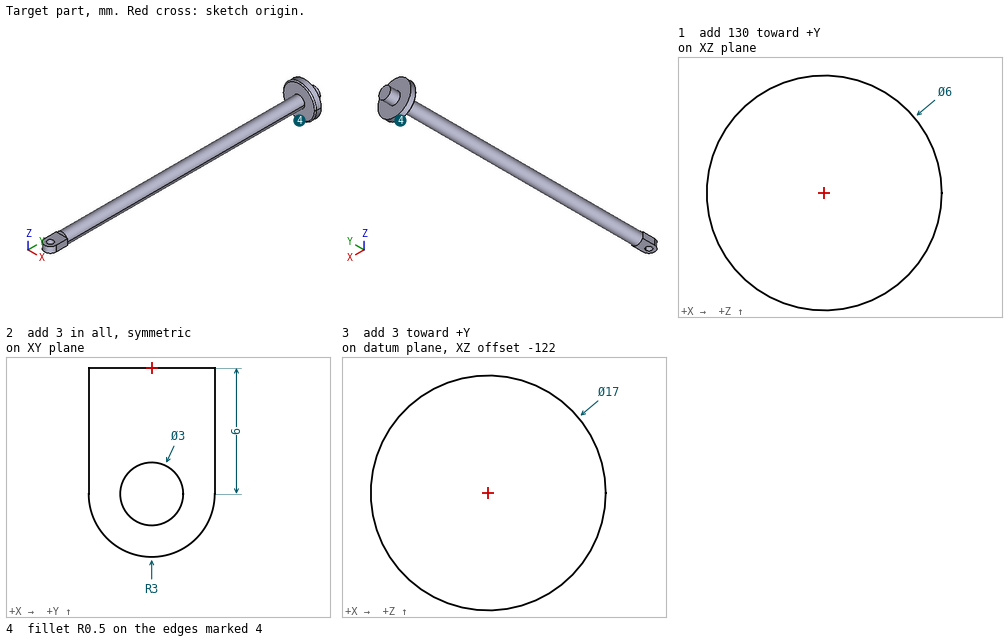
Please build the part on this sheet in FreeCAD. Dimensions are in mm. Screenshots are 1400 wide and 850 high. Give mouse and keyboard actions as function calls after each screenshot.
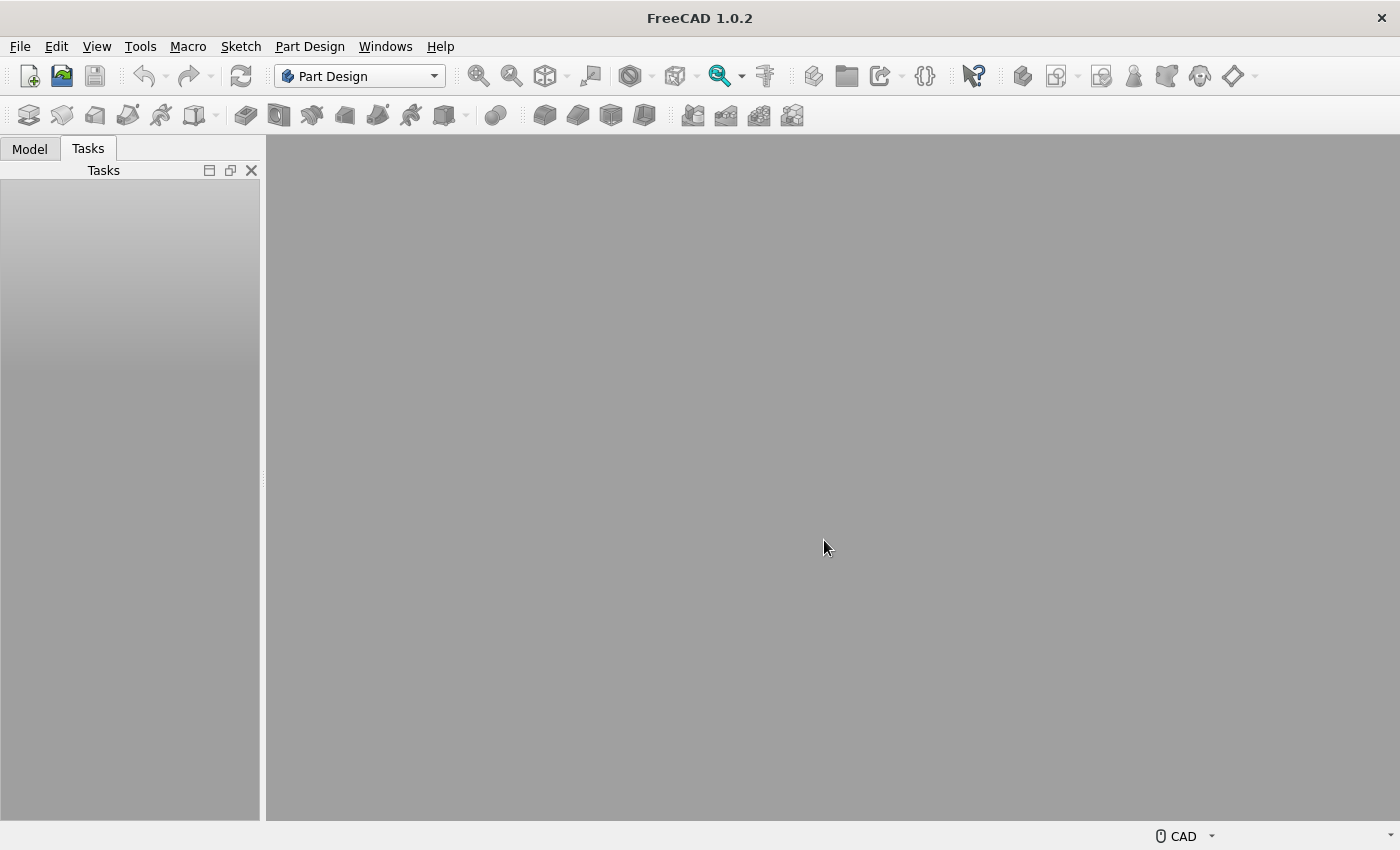
click(29, 76)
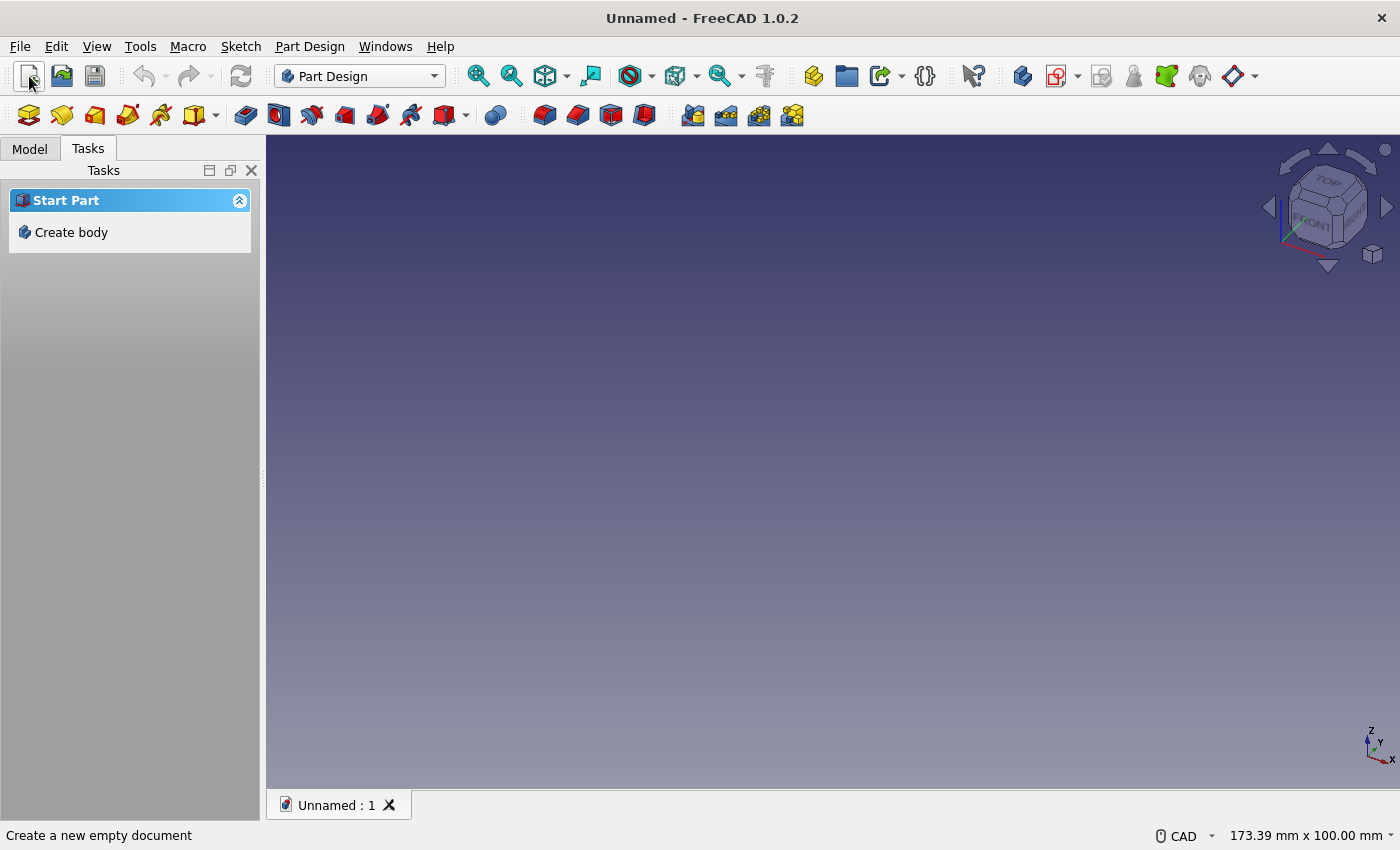
click(1056, 76)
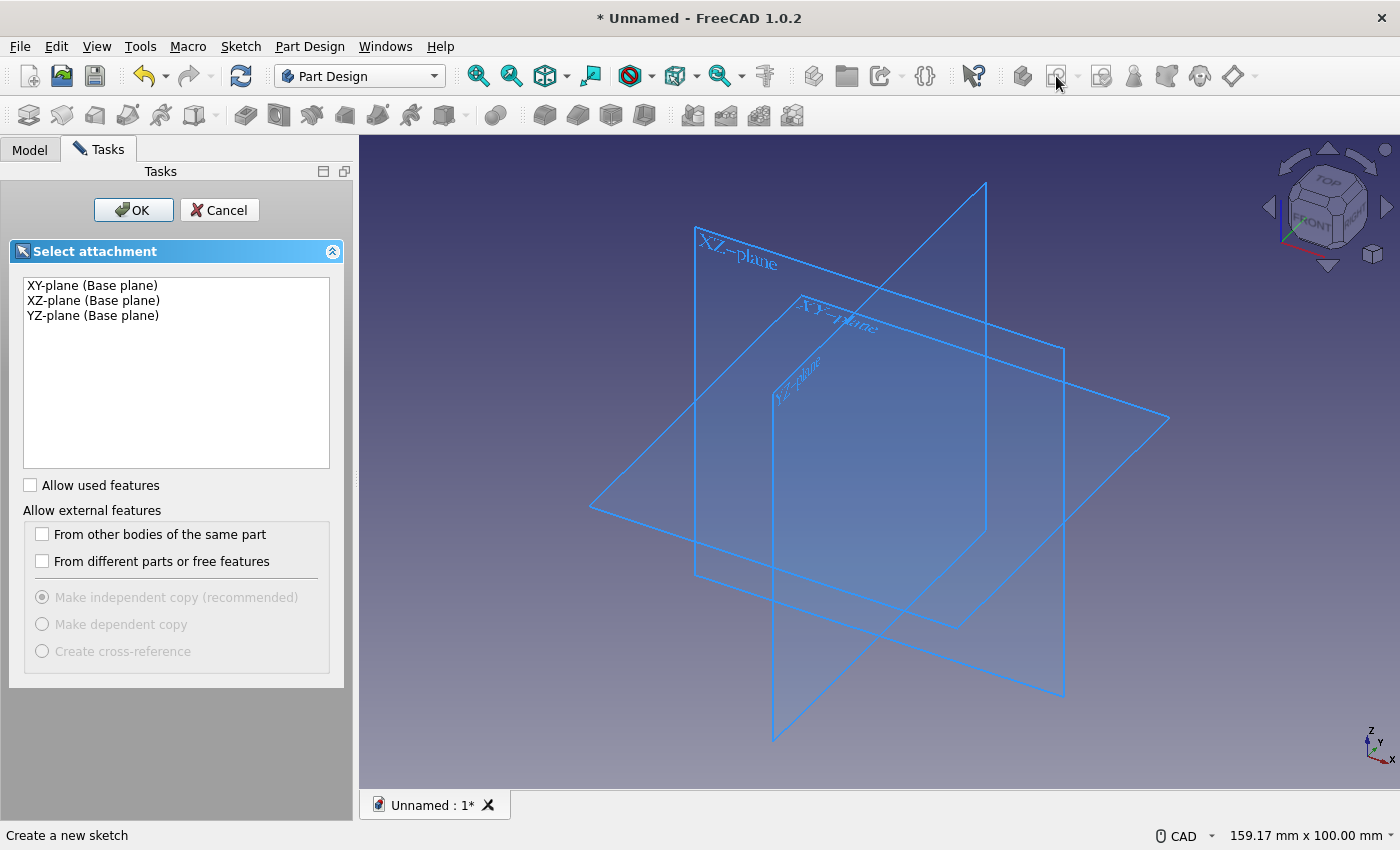
click(84, 300)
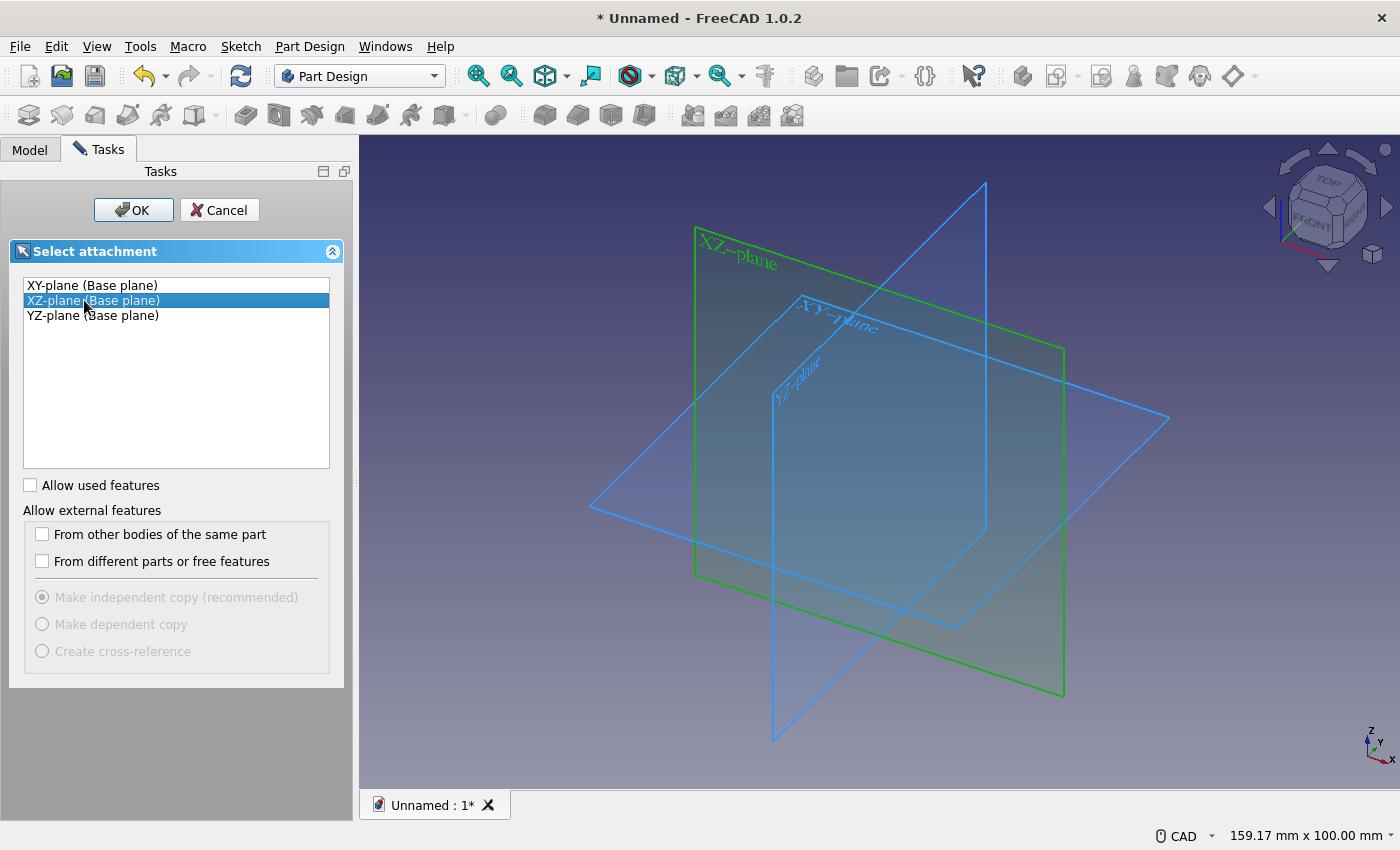
click(134, 210)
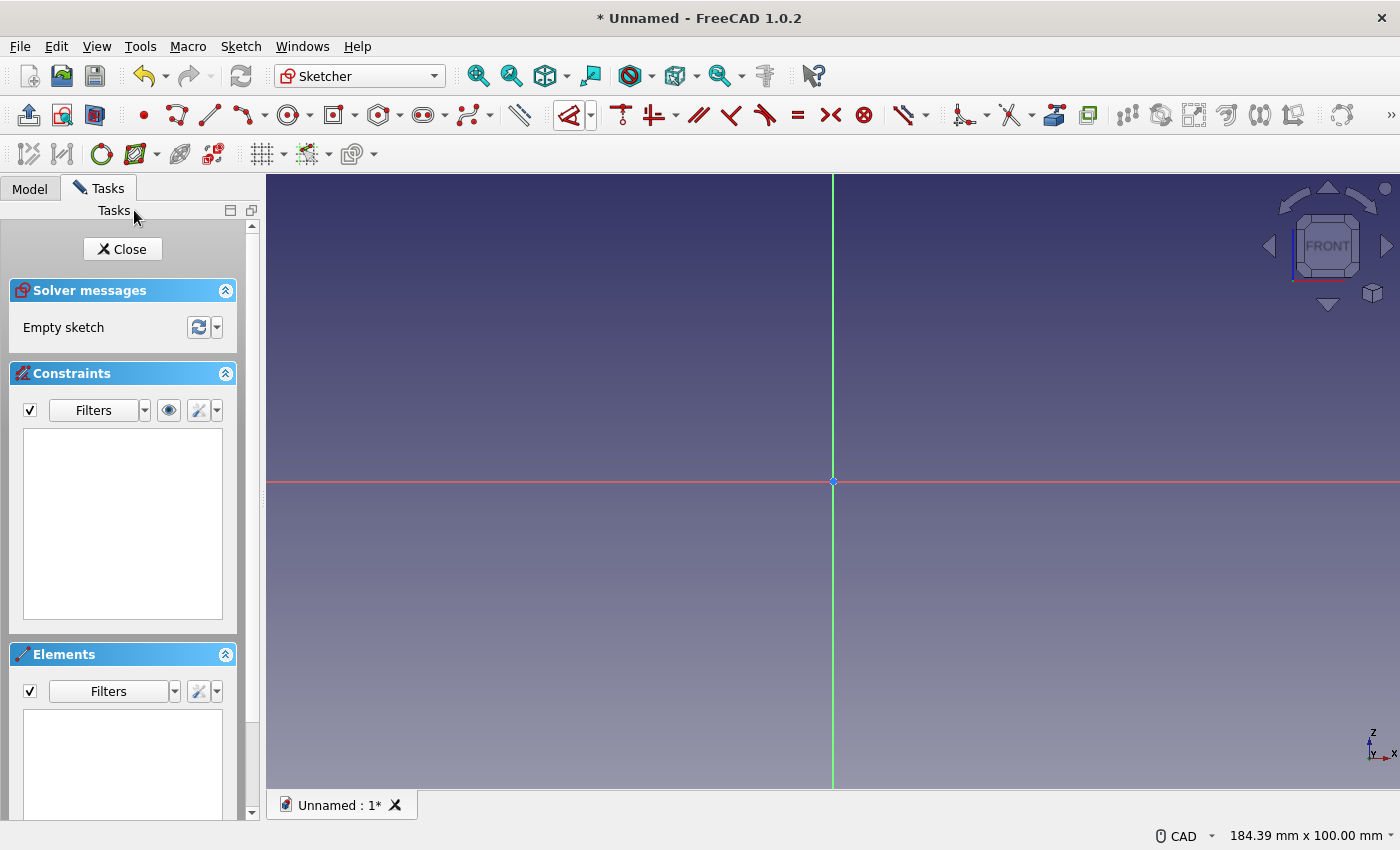
scroll(840, 482, up, 12)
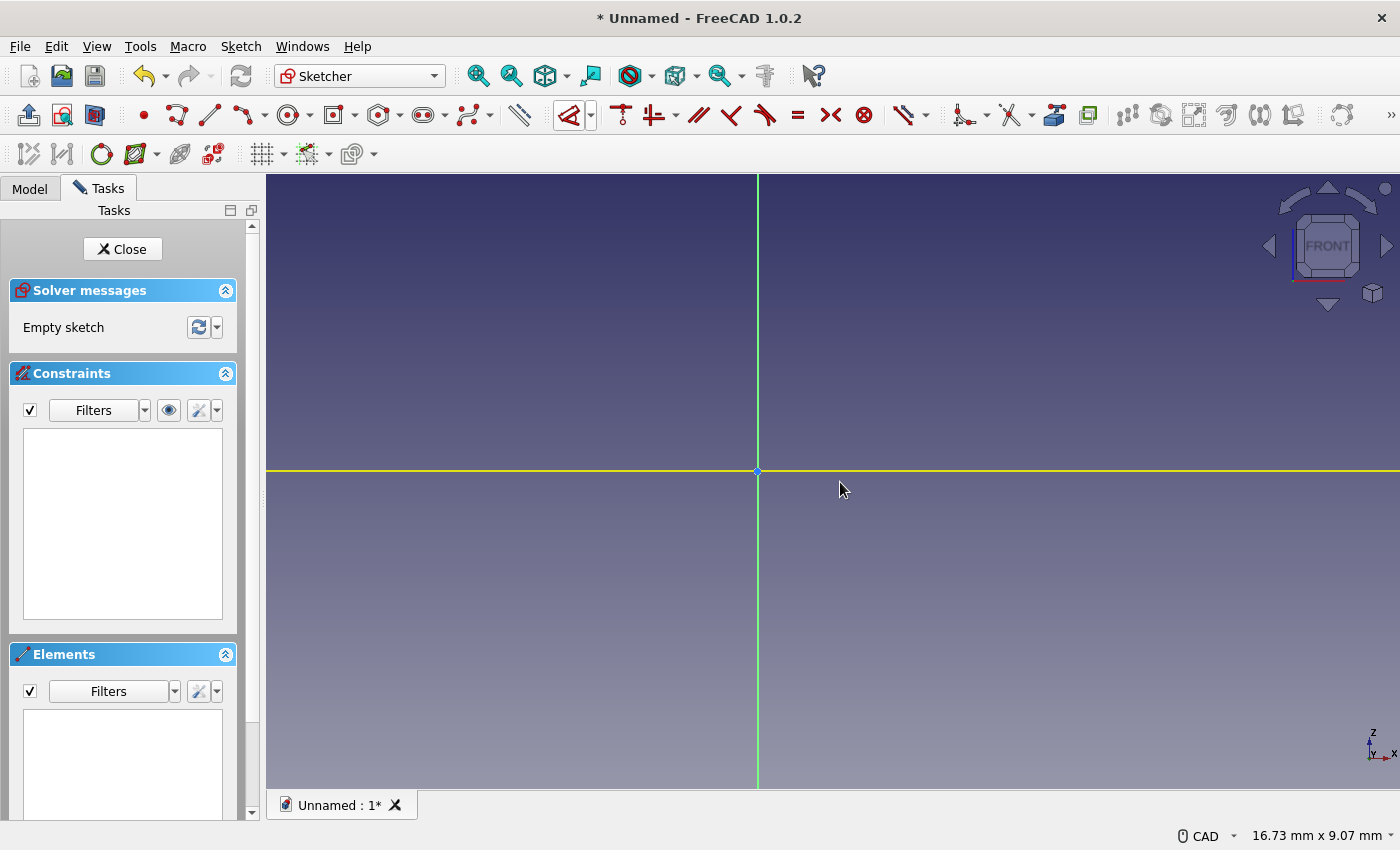
key(g)
key(c)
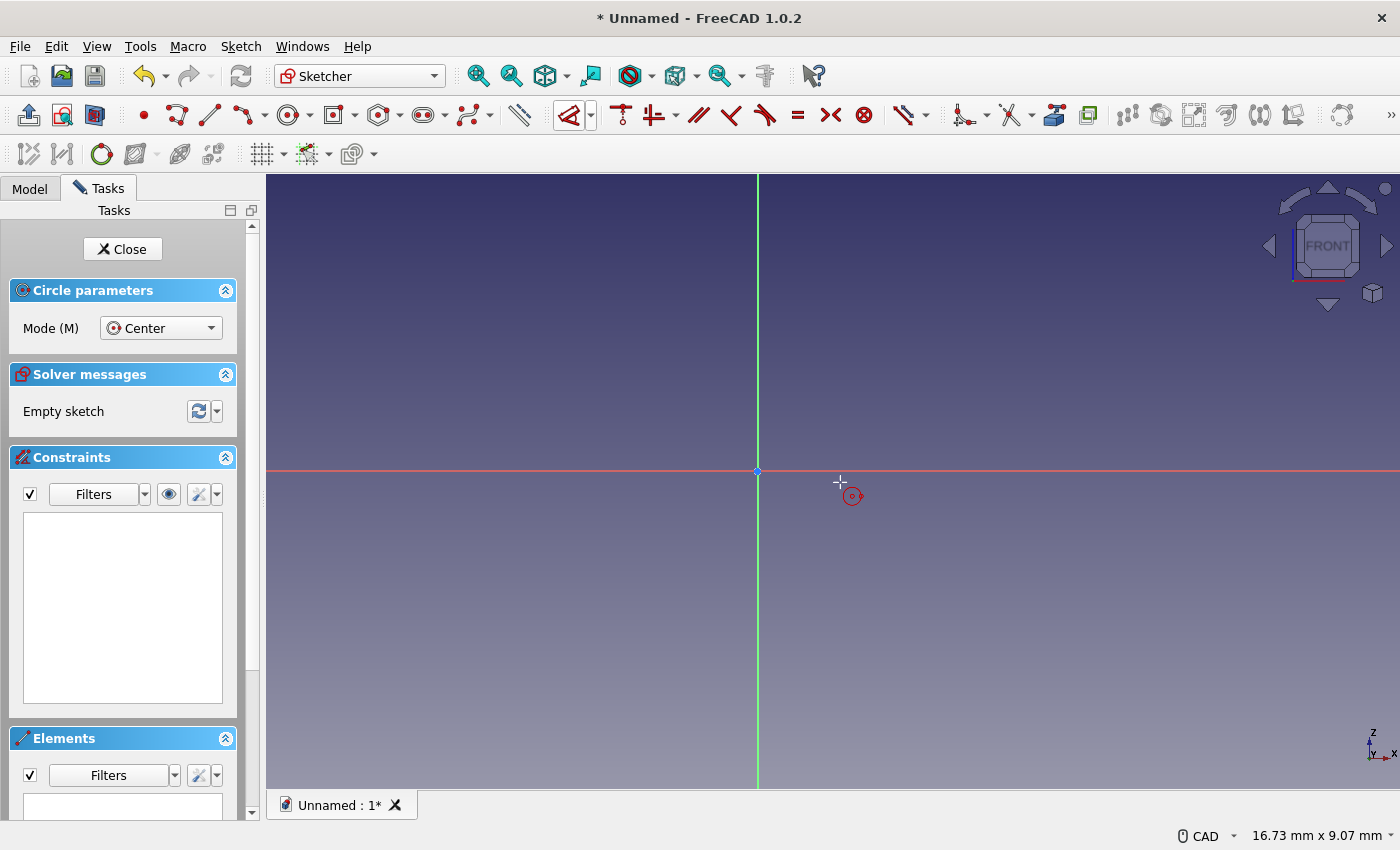
click(758, 471)
click(902, 328)
key(Escape)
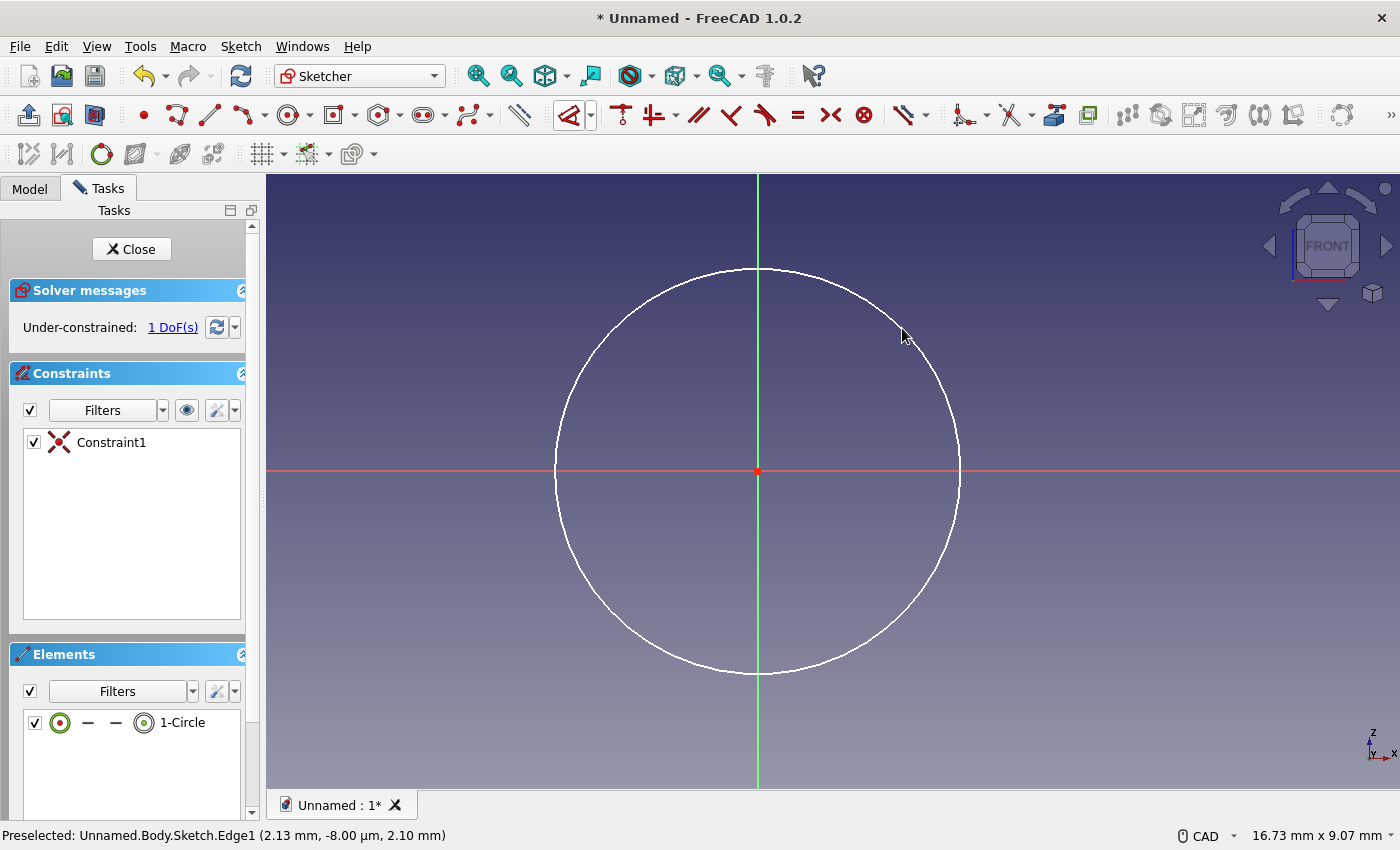
click(568, 116)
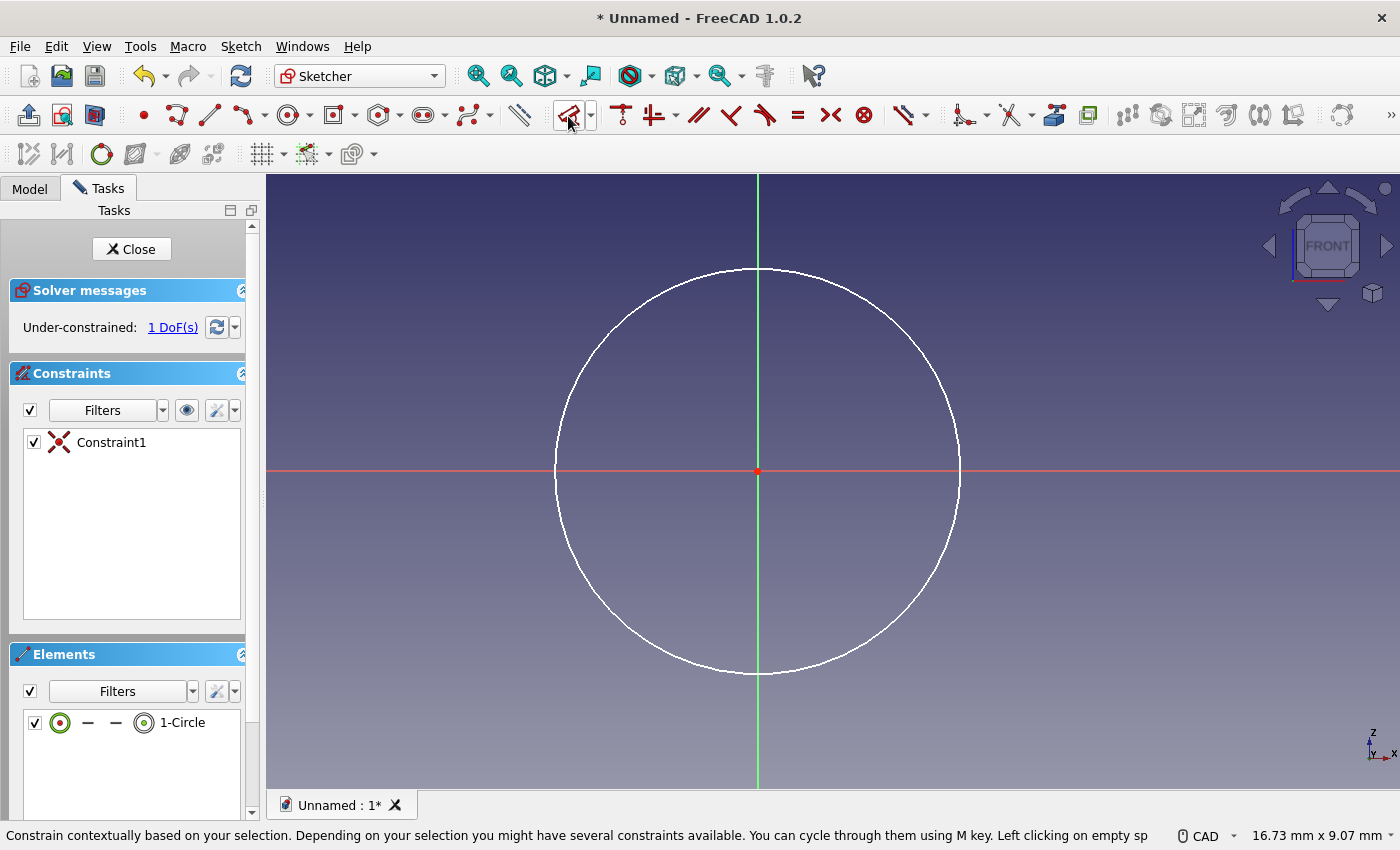
click(901, 328)
click(924, 305)